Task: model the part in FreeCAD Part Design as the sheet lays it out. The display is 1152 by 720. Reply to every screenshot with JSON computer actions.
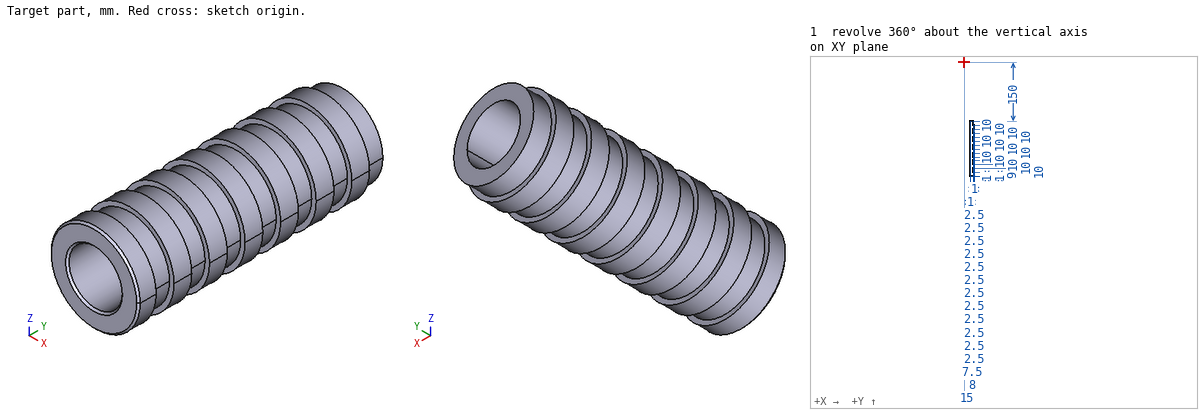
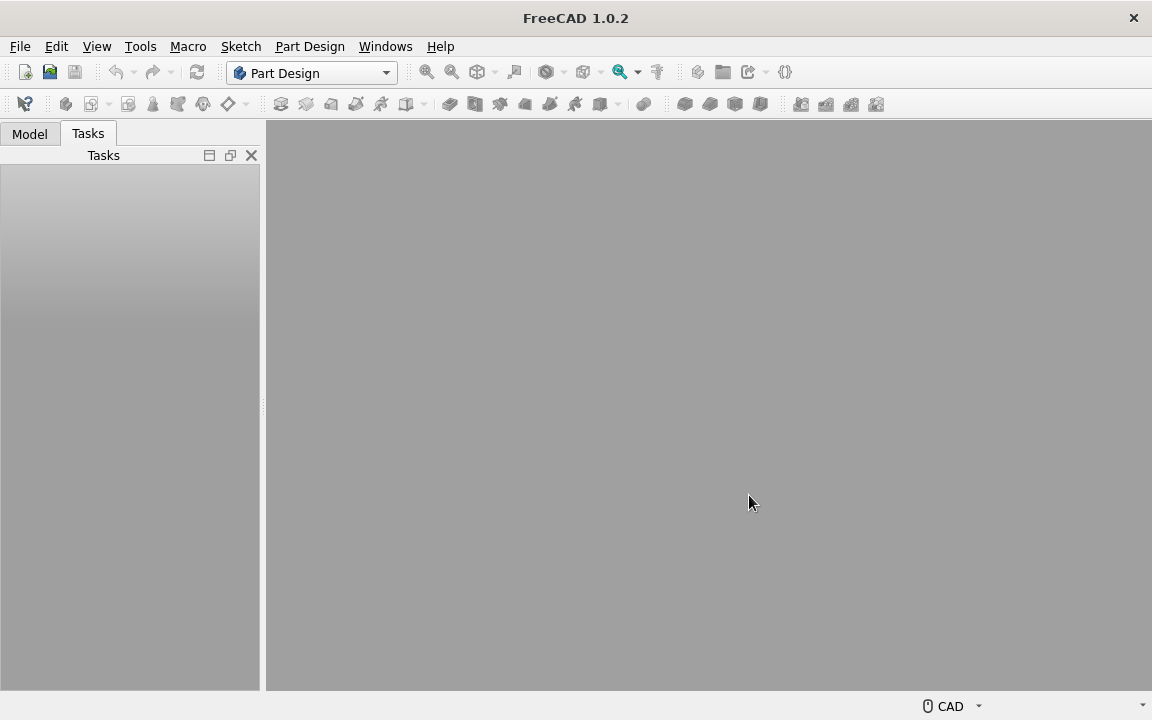
{"action": "key", "text": "ctrl+n"}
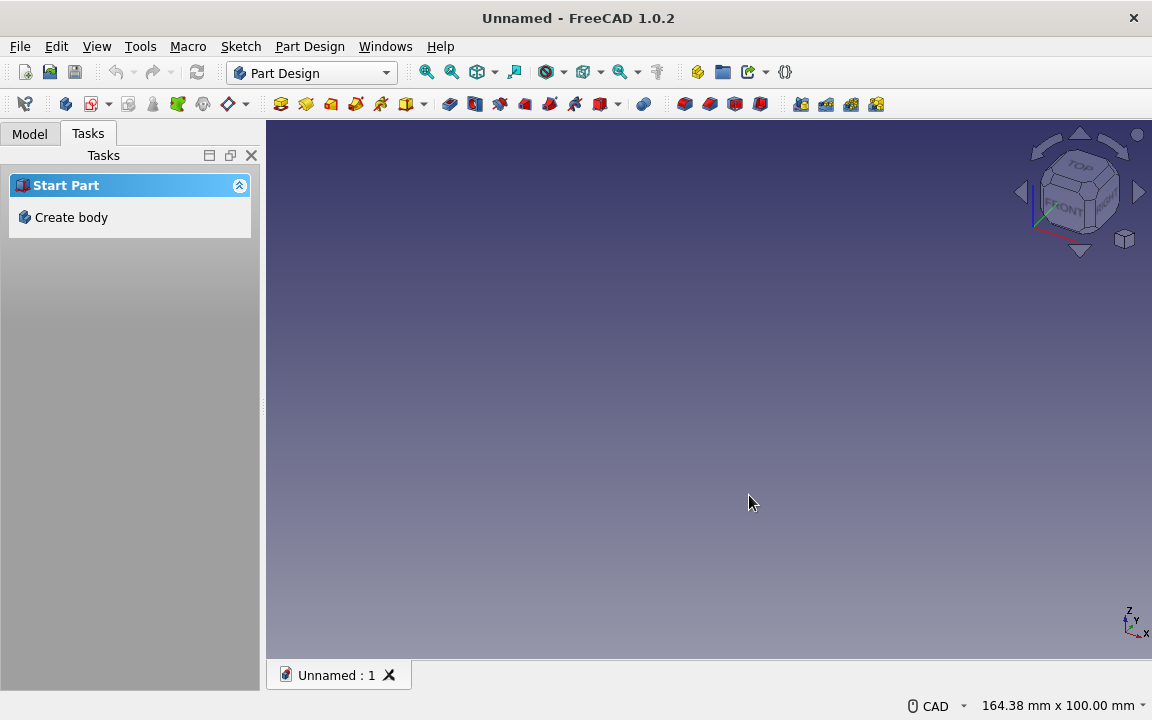
{"action": "left_click", "coordinate": [90, 104]}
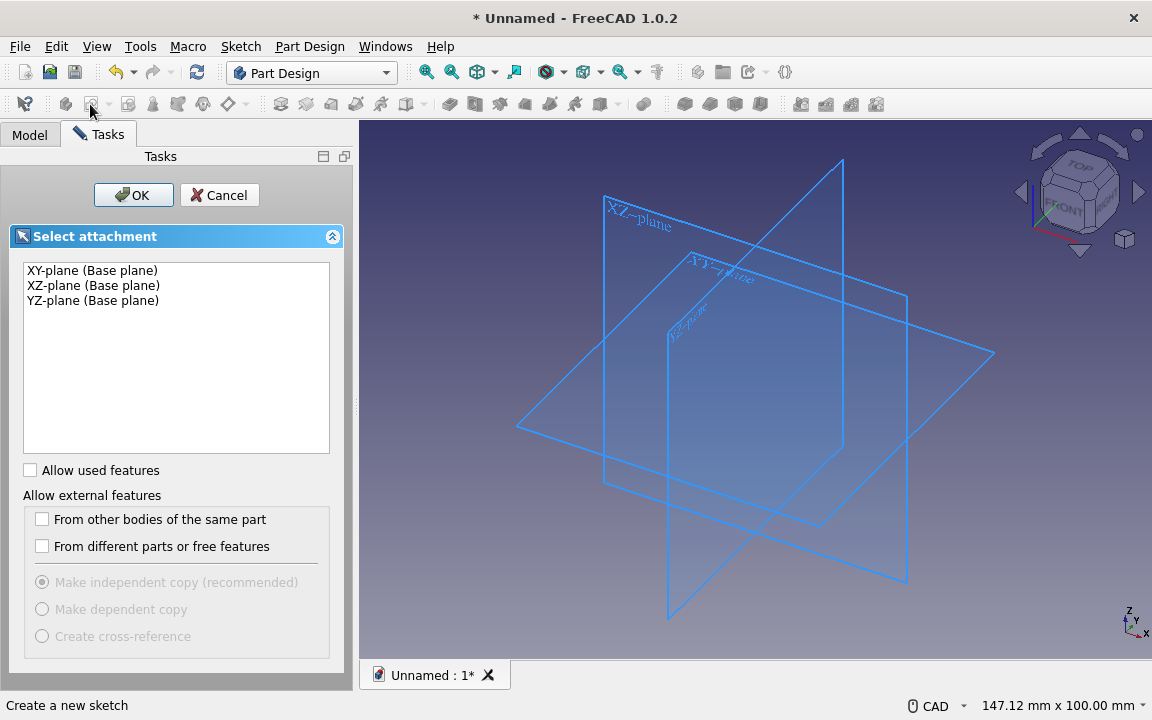
{"action": "left_click", "coordinate": [84, 270]}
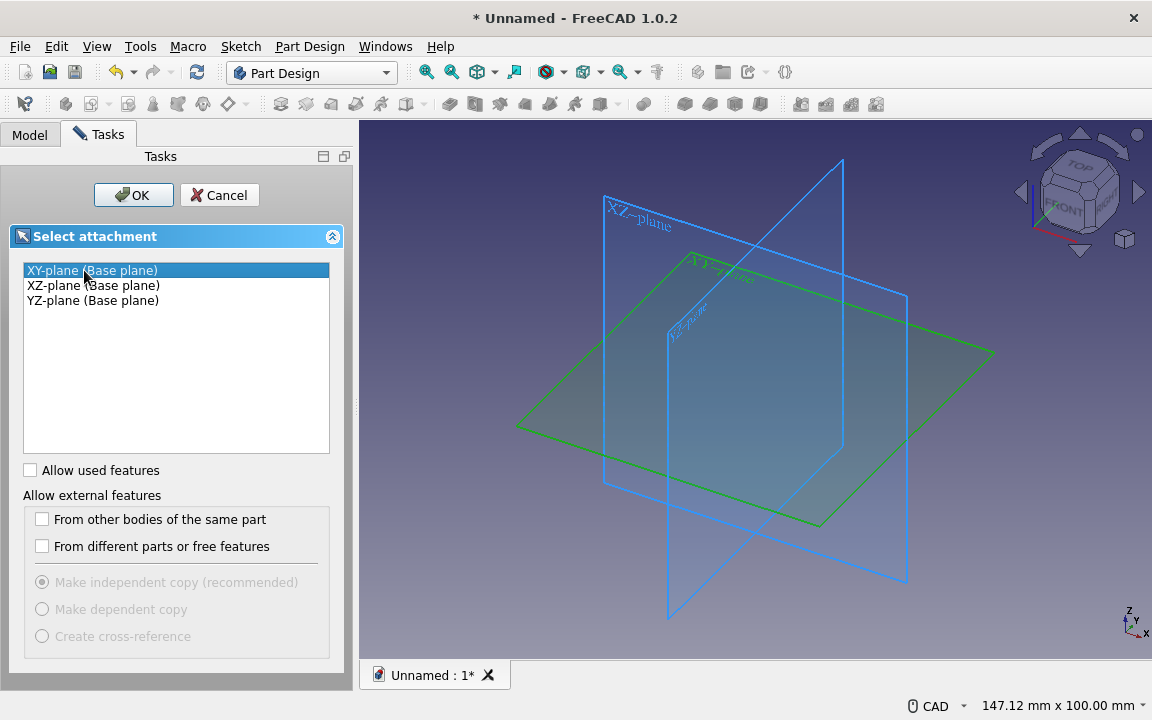
{"action": "left_click", "coordinate": [134, 195]}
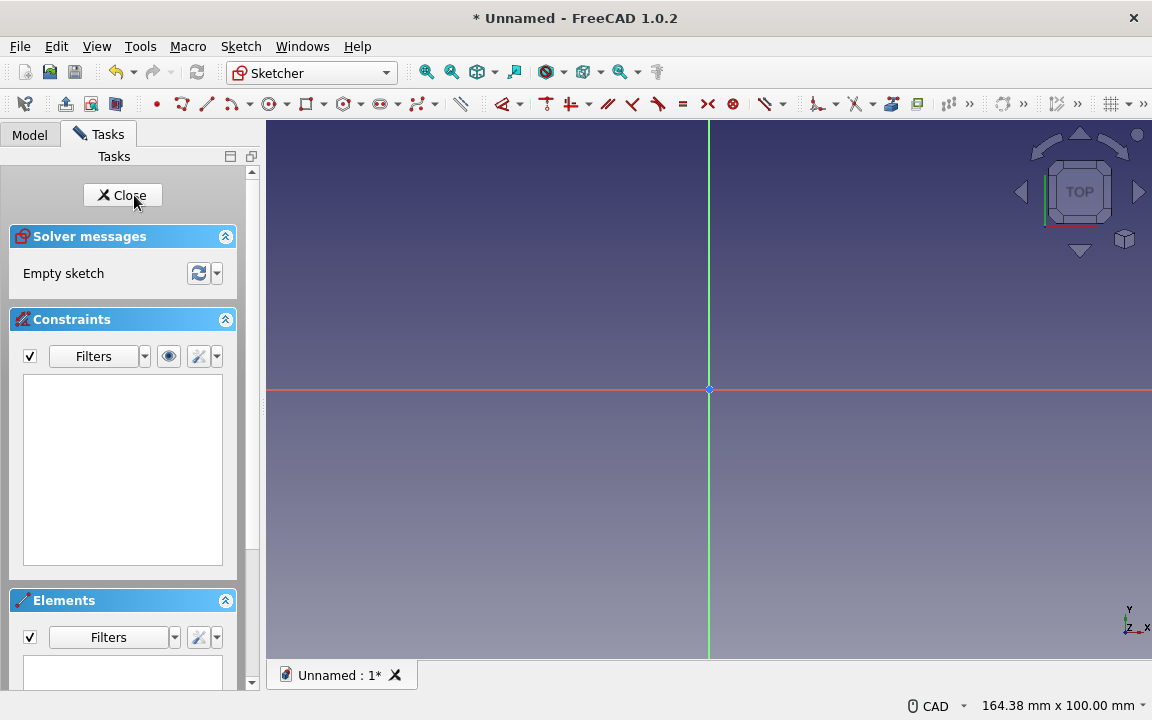
{"action": "scroll", "coordinate": [606, 192], "scroll_direction": "down", "scroll_amount": 8}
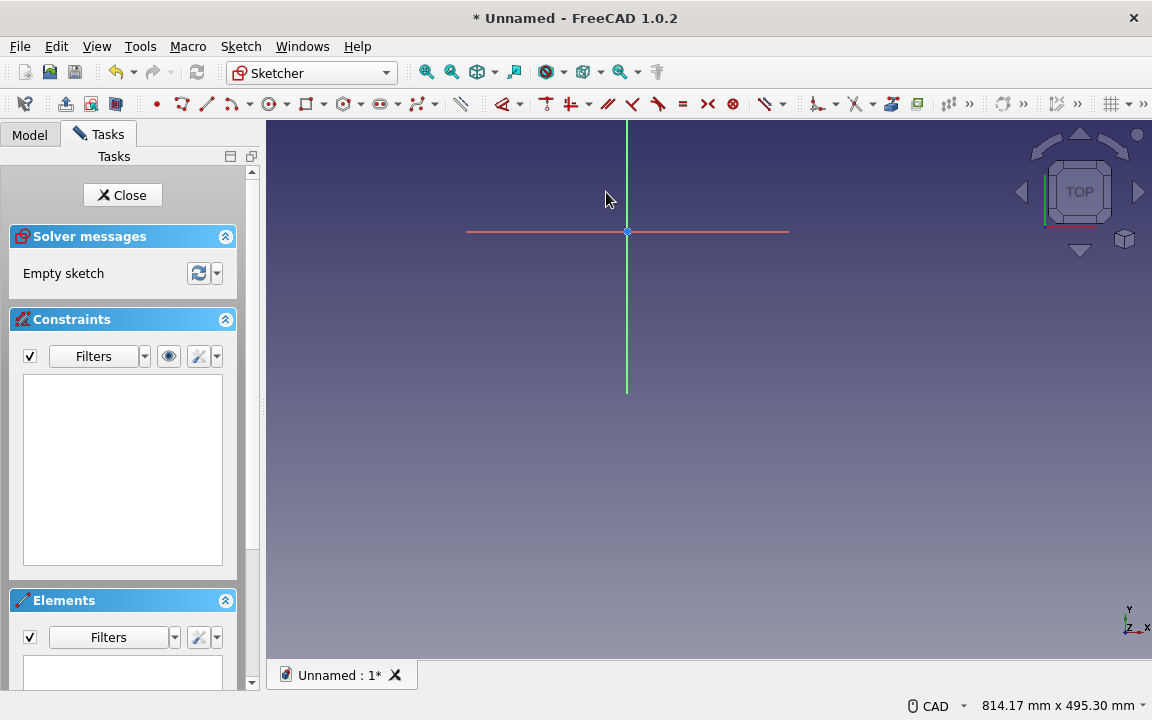
{"action": "key", "text": "g m"}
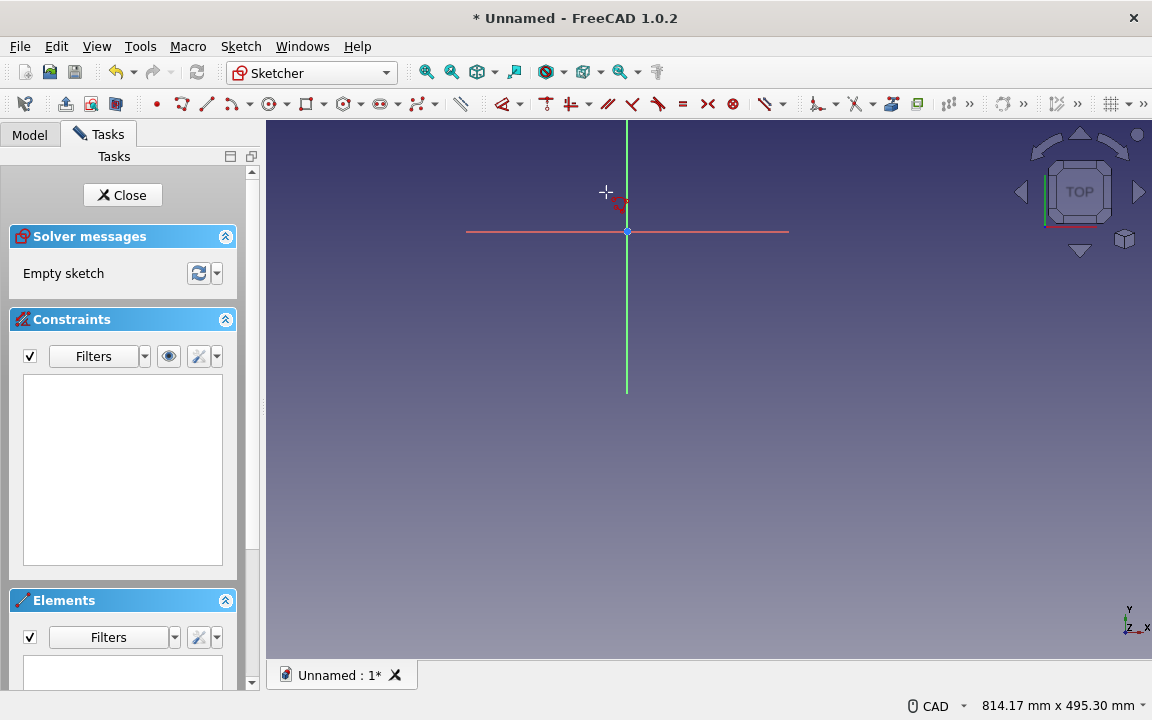
{"action": "left_click", "coordinate": [643, 395]}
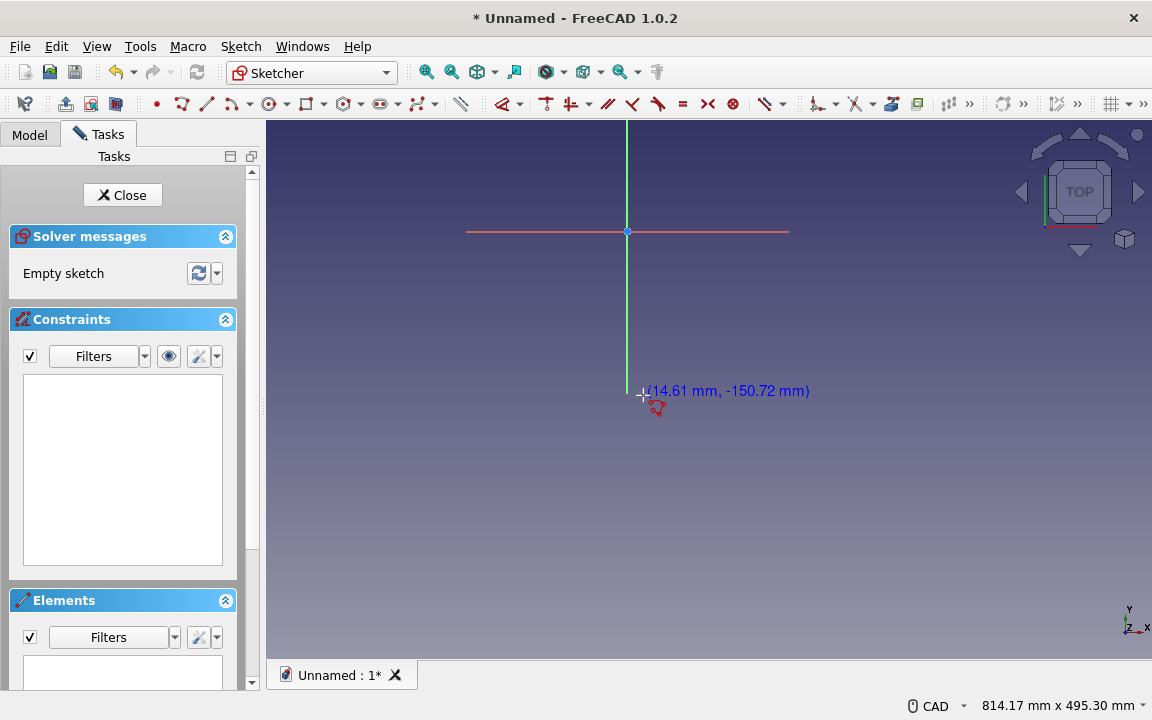
{"action": "scroll", "coordinate": [652, 395], "scroll_direction": "up", "scroll_amount": 4}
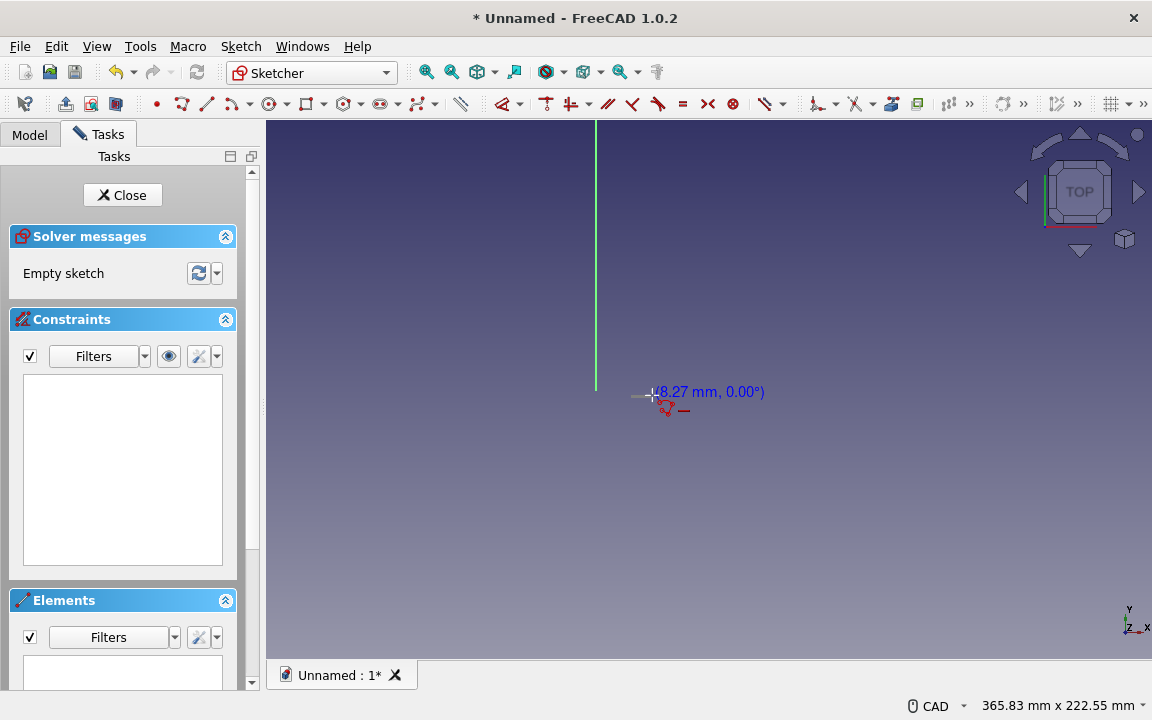
{"action": "left_click", "coordinate": [651, 394]}
{"action": "left_click", "coordinate": [651, 419]}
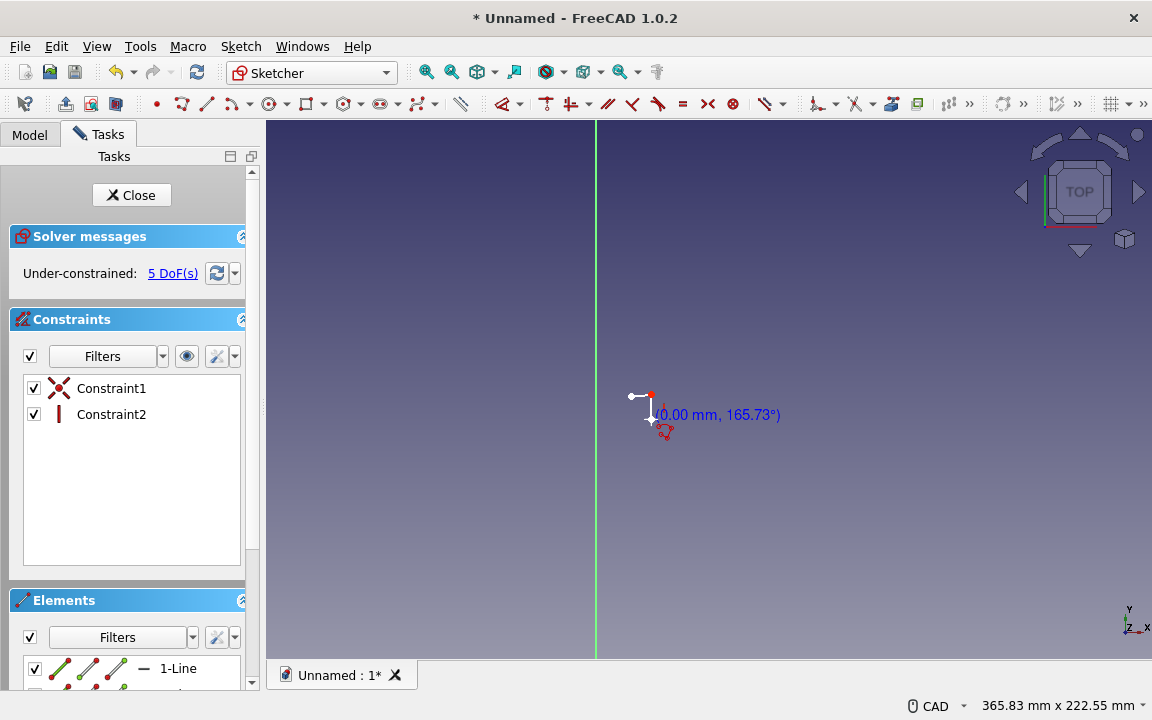
{"action": "scroll", "coordinate": [657, 419], "scroll_direction": "up", "scroll_amount": 5}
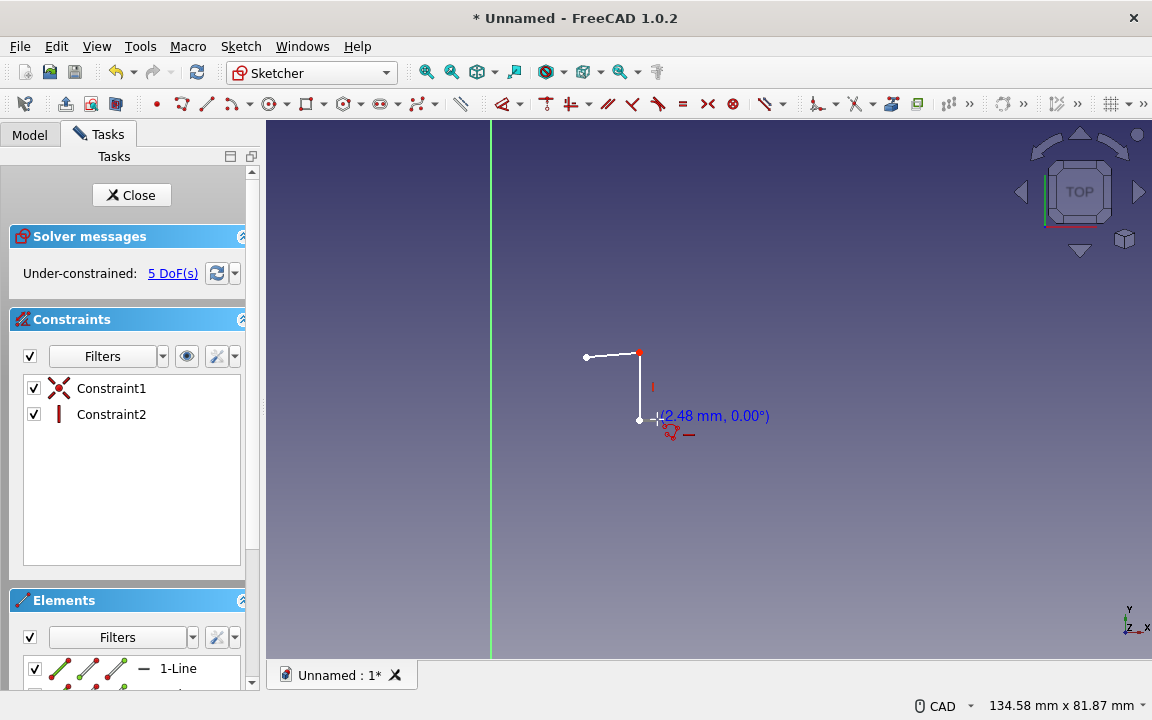
{"action": "left_click", "coordinate": [655, 418]}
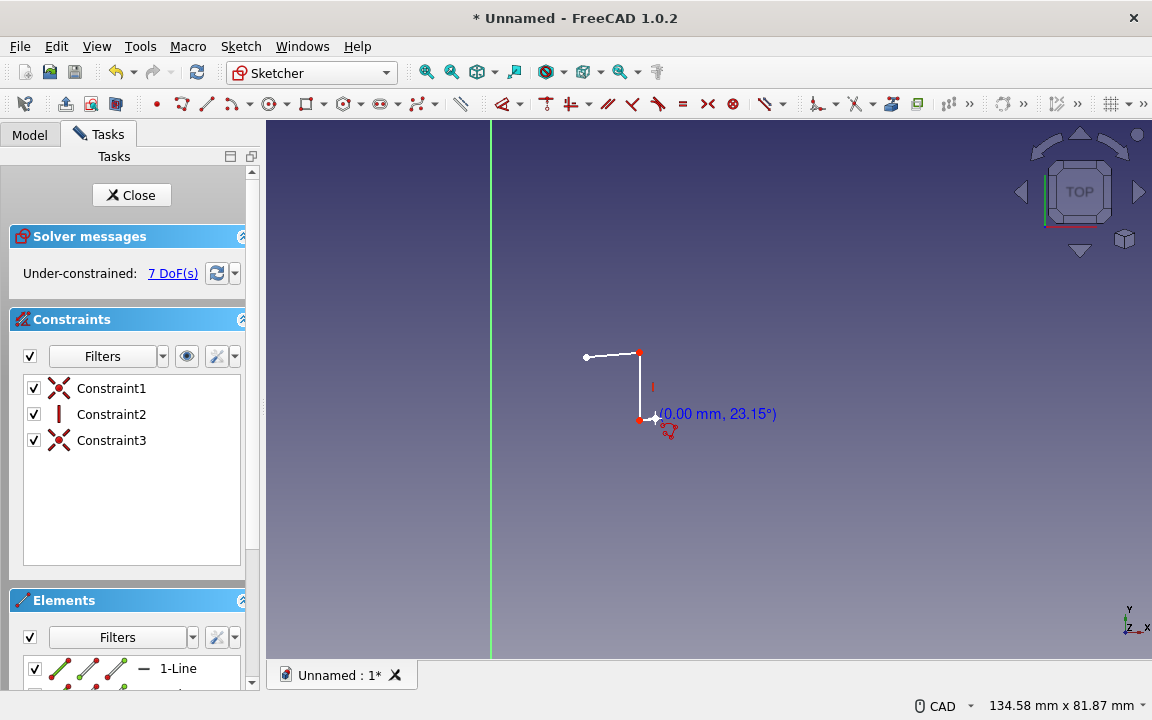
{"action": "scroll", "coordinate": [654, 403], "scroll_direction": "down", "scroll_amount": 9}